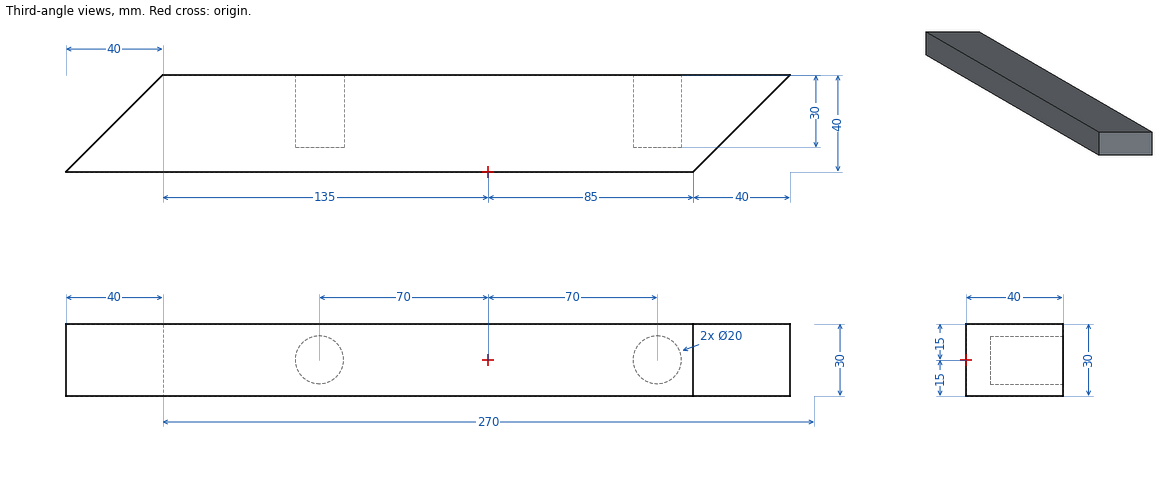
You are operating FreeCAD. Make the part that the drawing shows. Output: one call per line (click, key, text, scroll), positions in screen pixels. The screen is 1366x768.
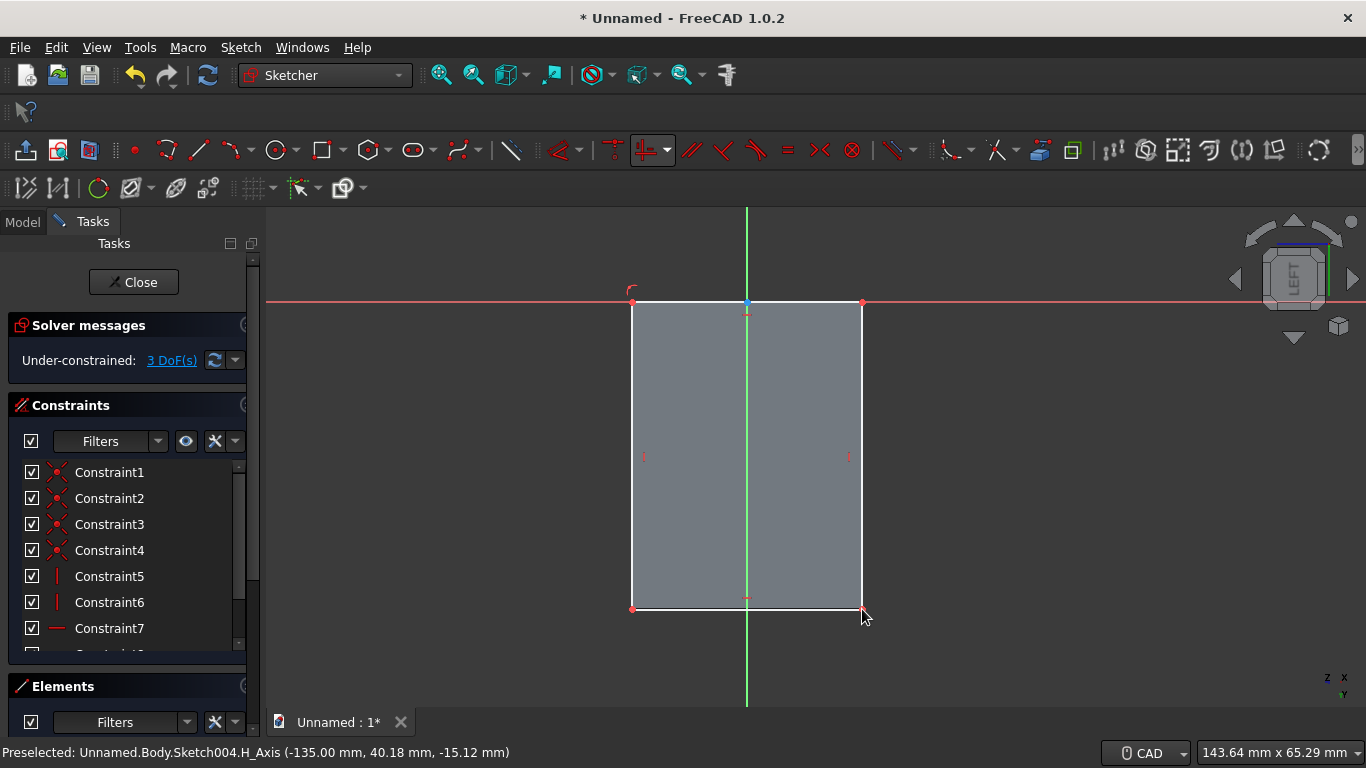
key(d)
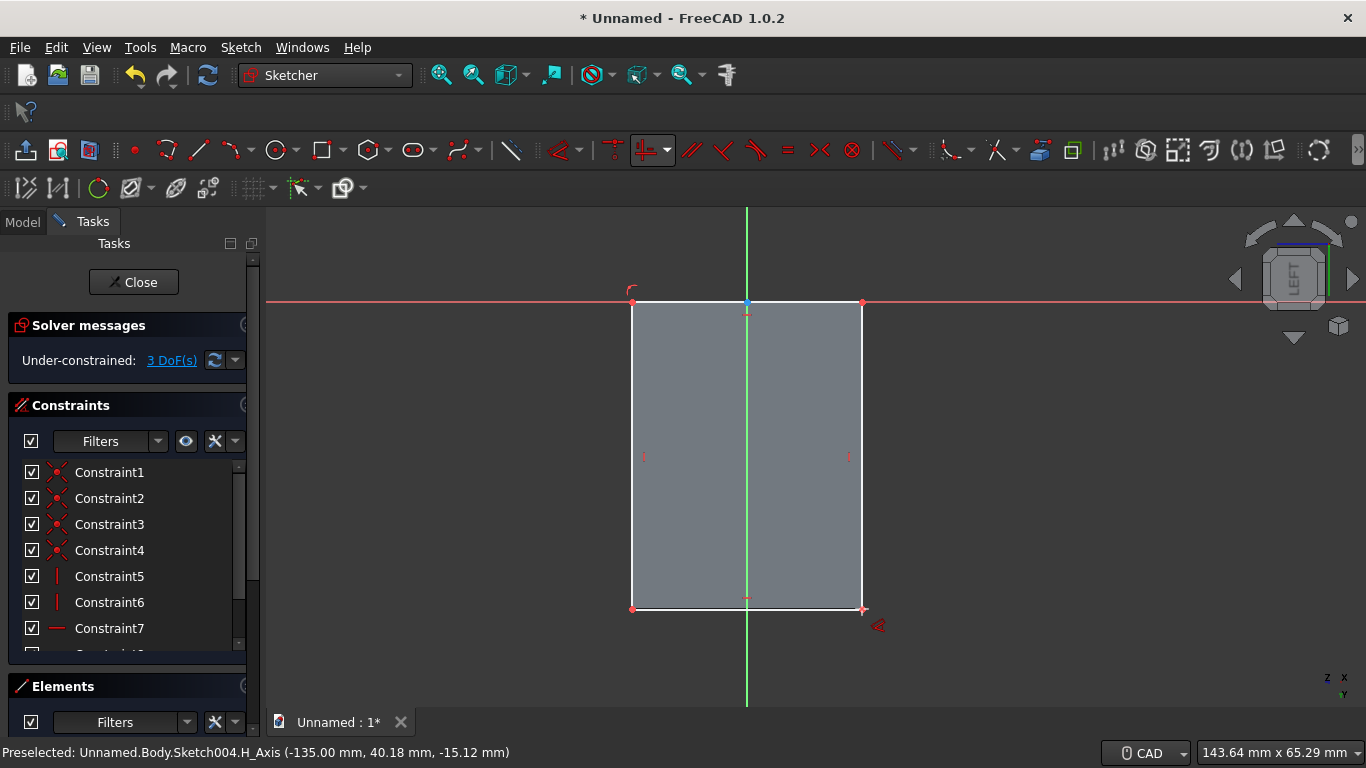
click(632, 395)
click(598, 456)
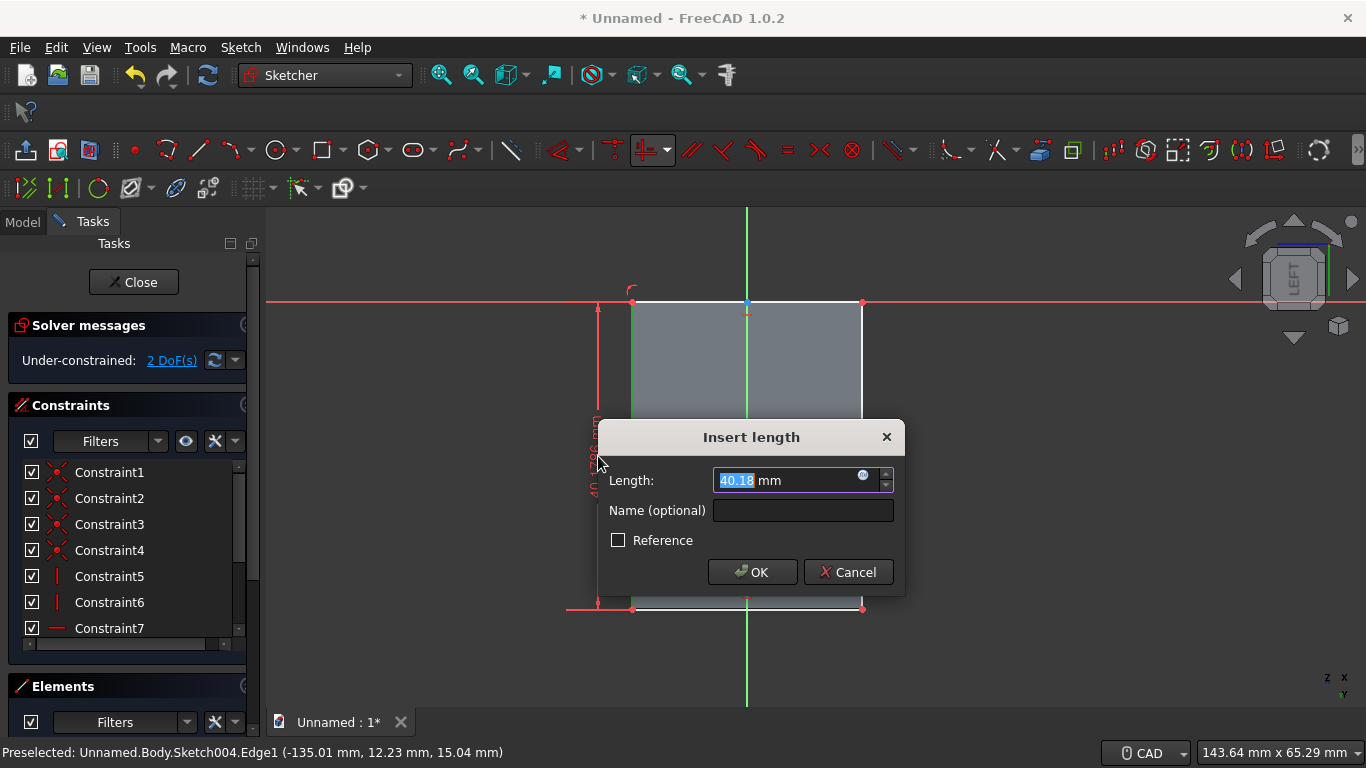
text(40)
key(Return)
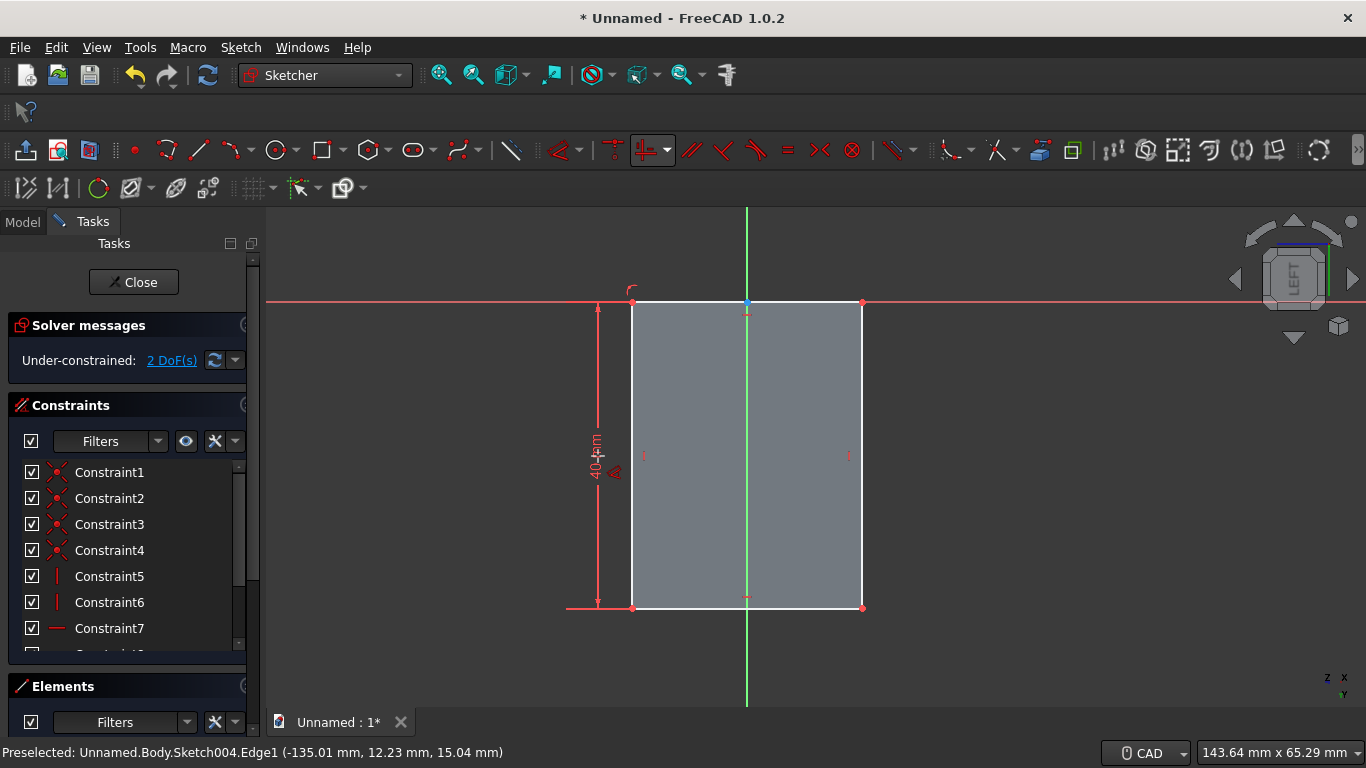
click(701, 609)
click(694, 643)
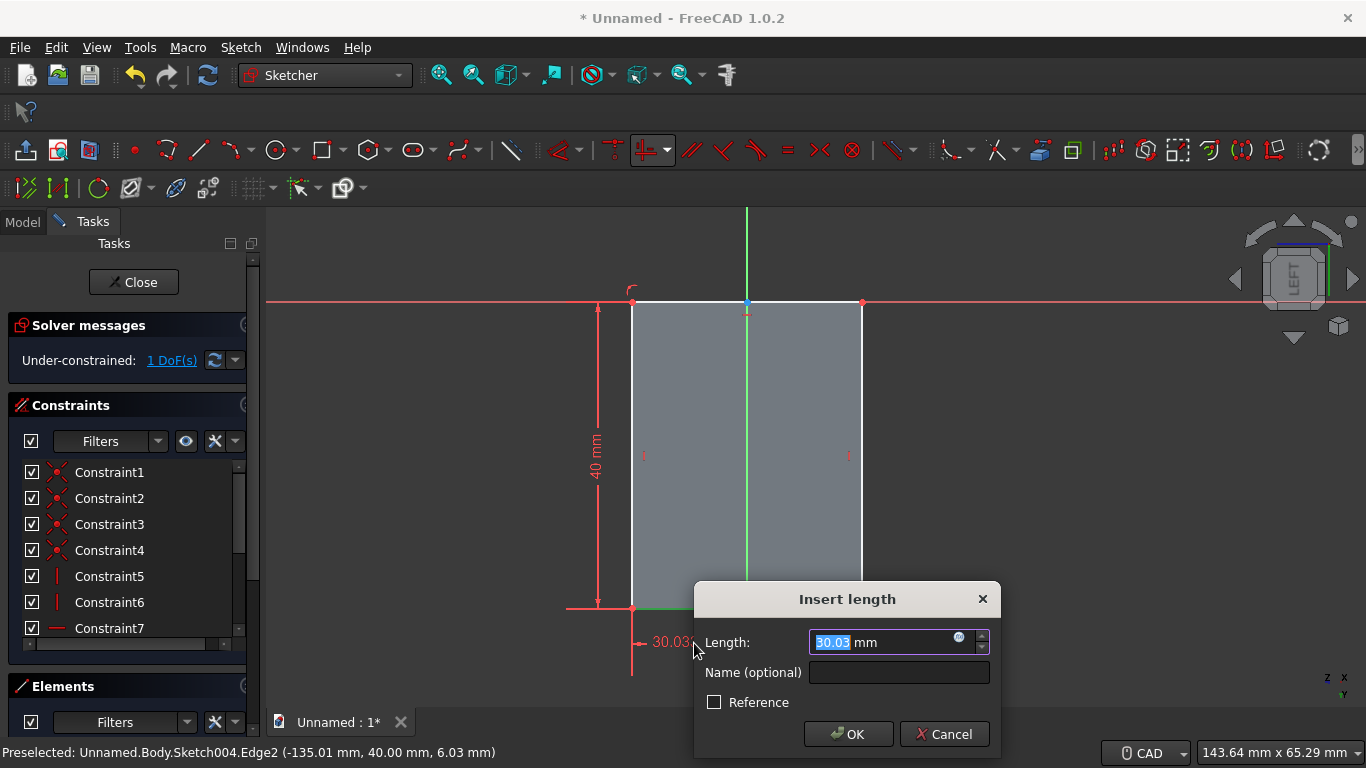
text(30)
key(Return)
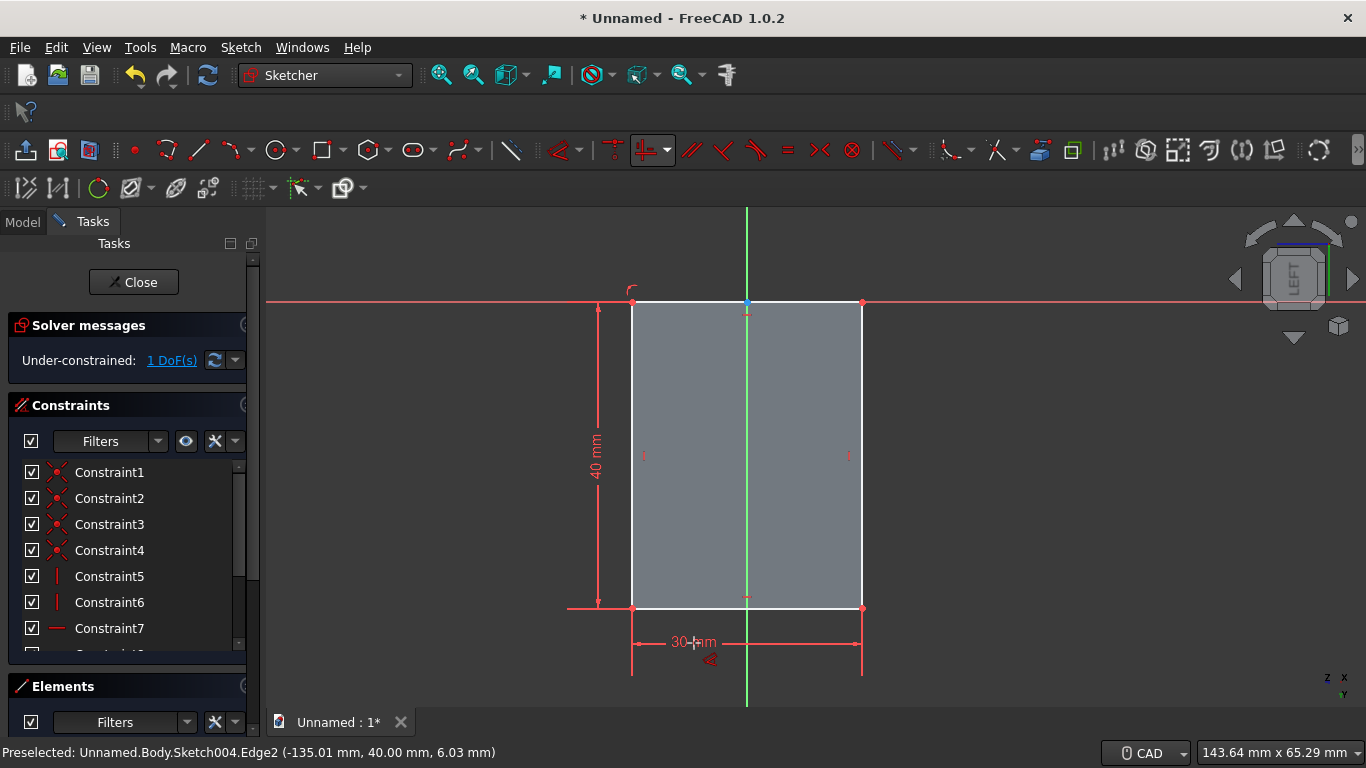
click(632, 302)
click(690, 268)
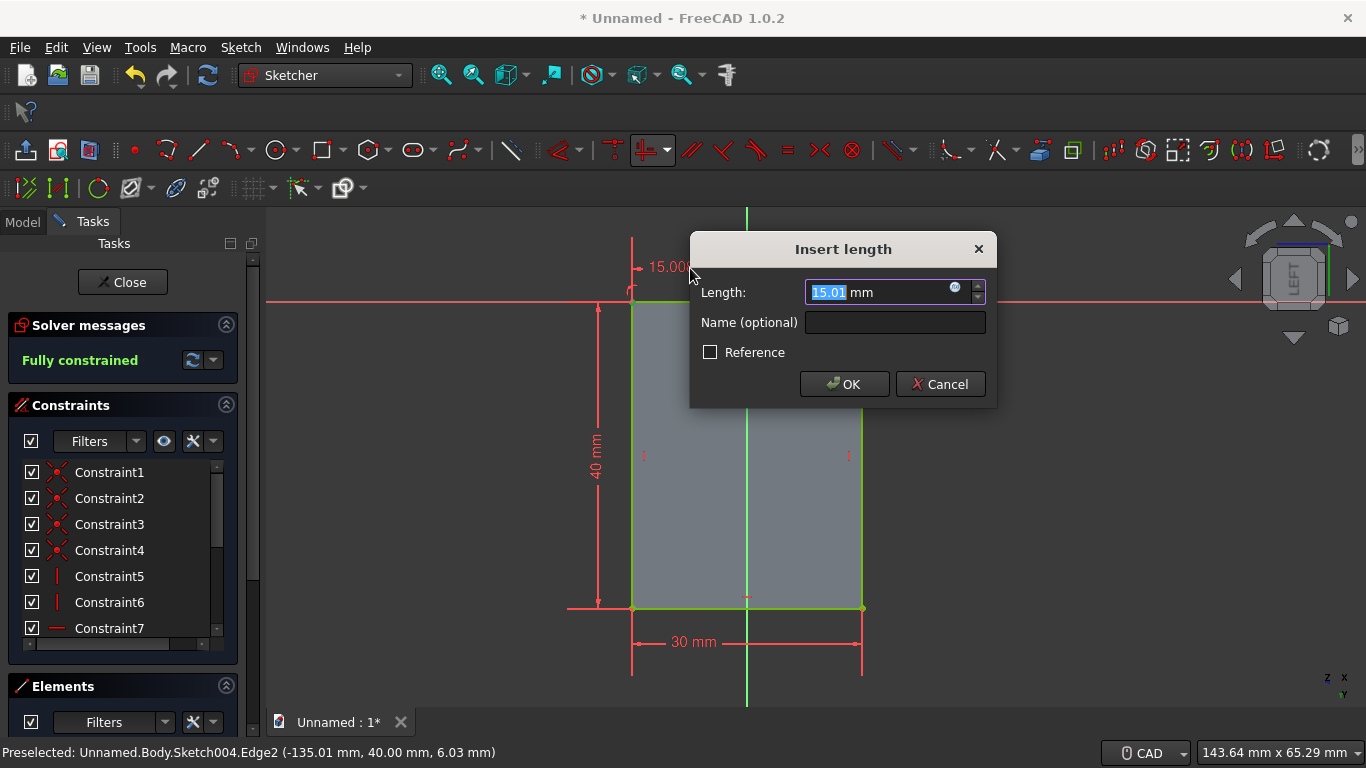
text(15)
key(Return)
key(Escape)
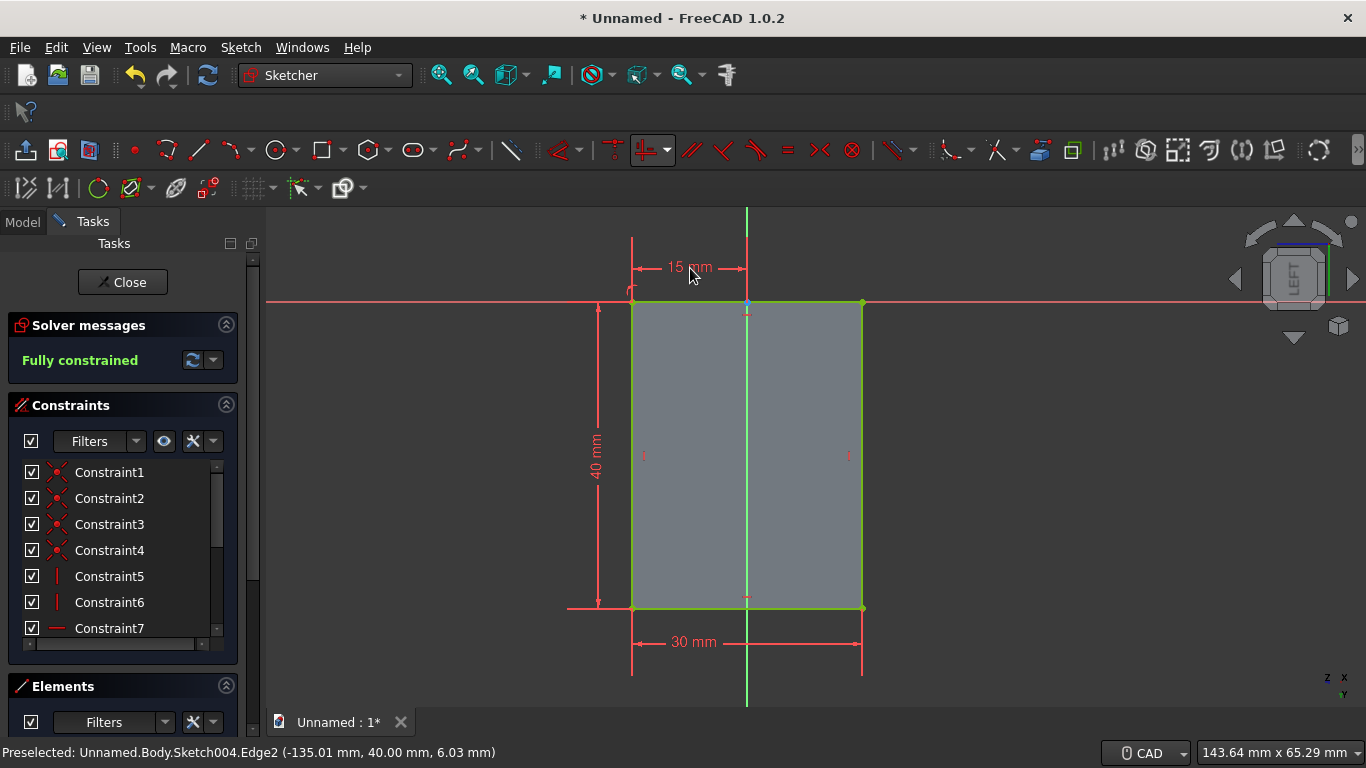
click(123, 282)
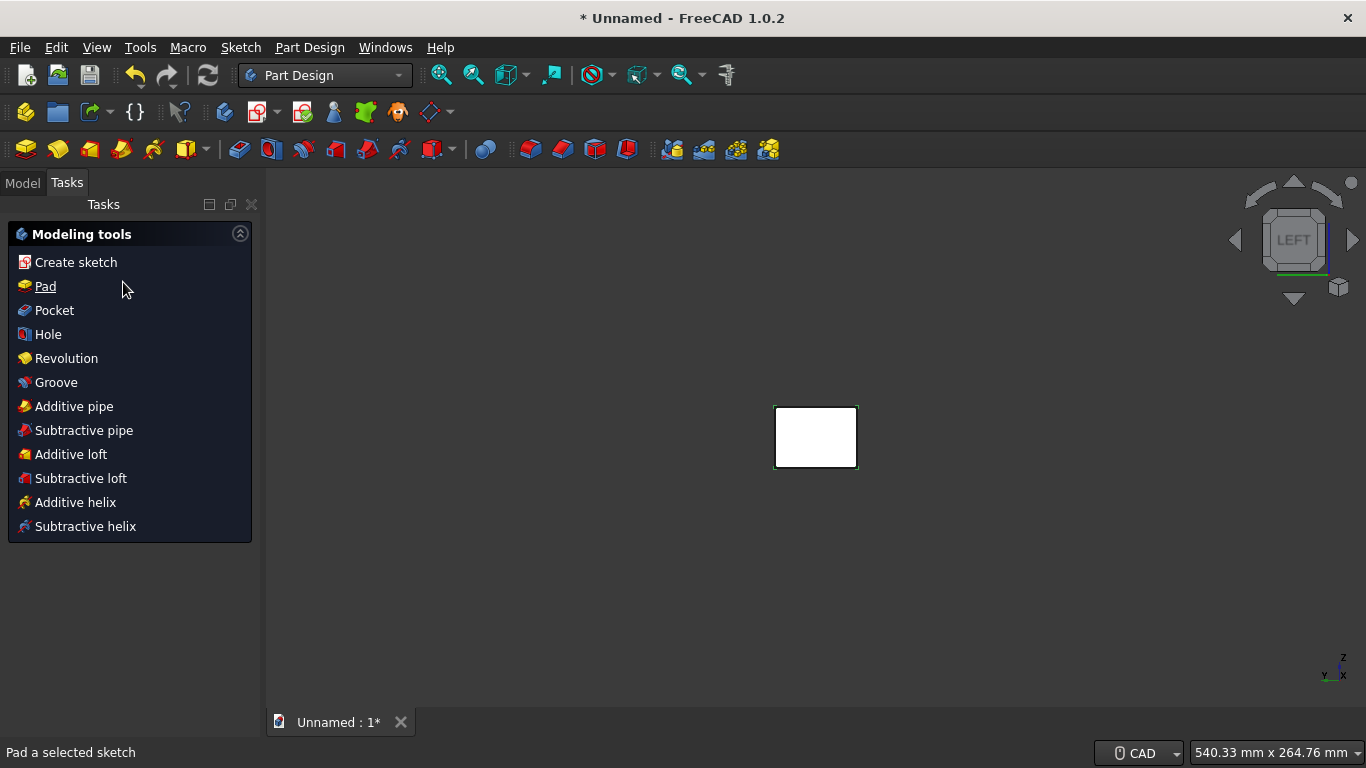
click(26, 150)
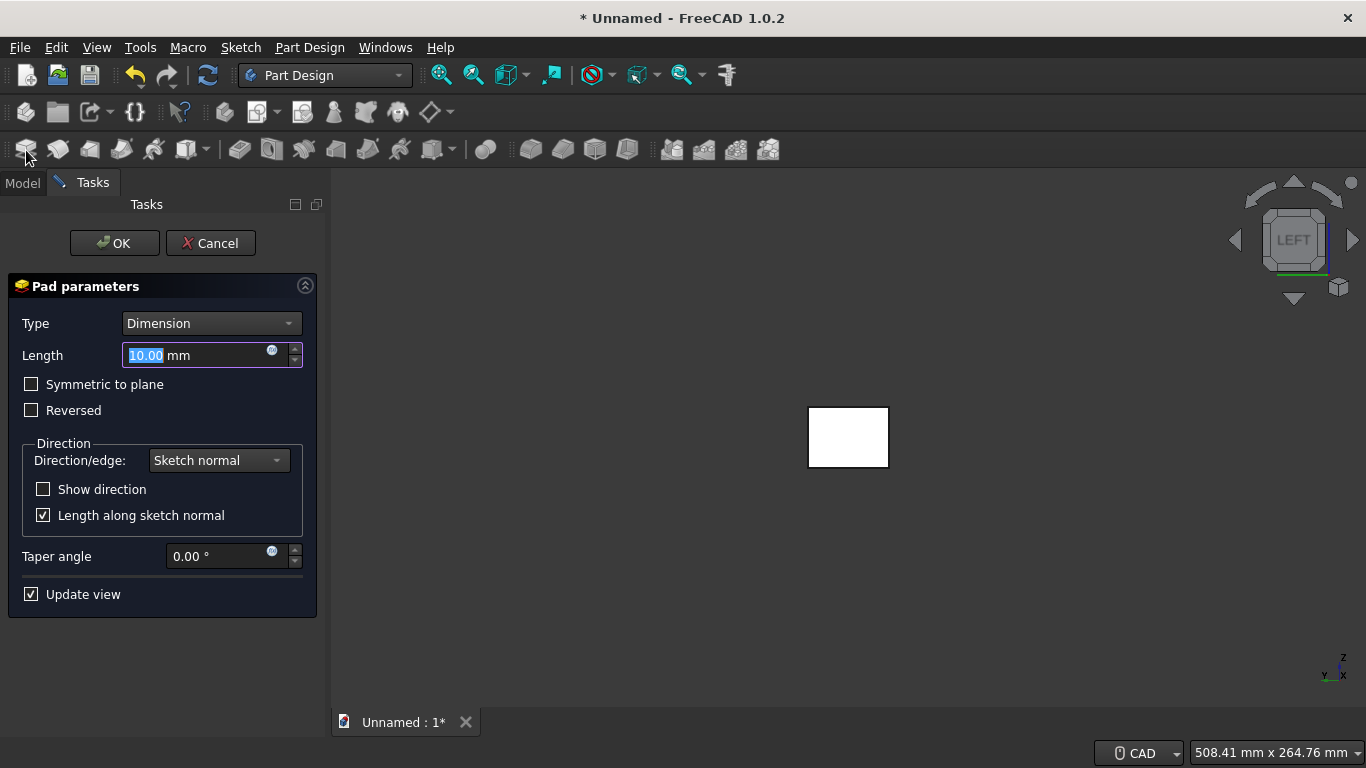
text(40)
key(Tab)